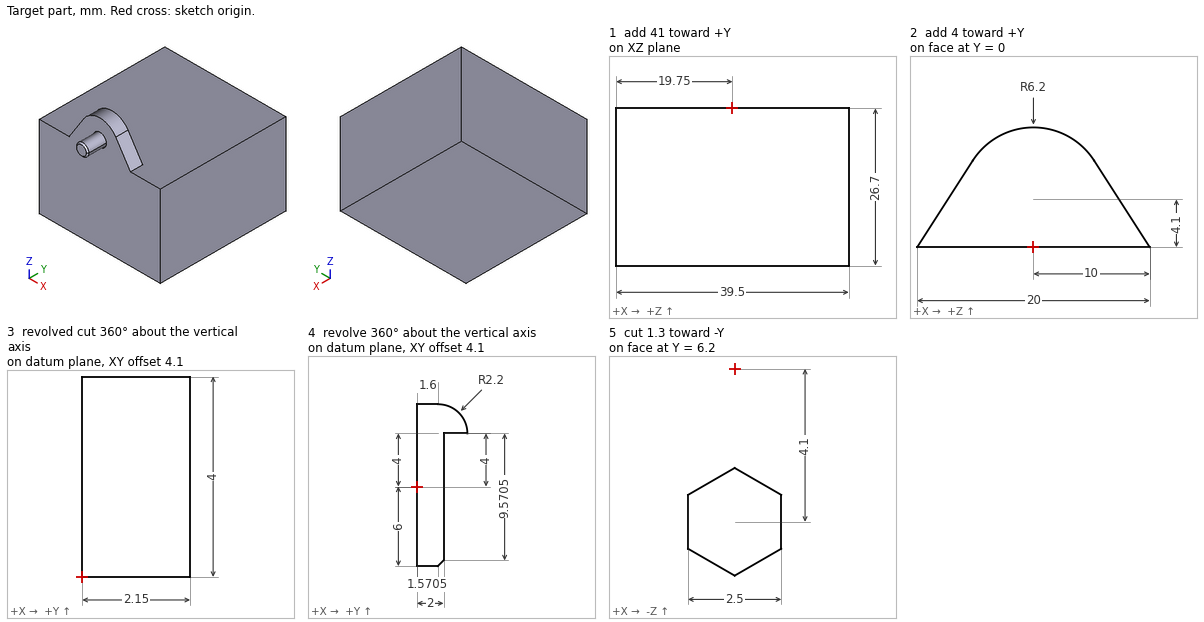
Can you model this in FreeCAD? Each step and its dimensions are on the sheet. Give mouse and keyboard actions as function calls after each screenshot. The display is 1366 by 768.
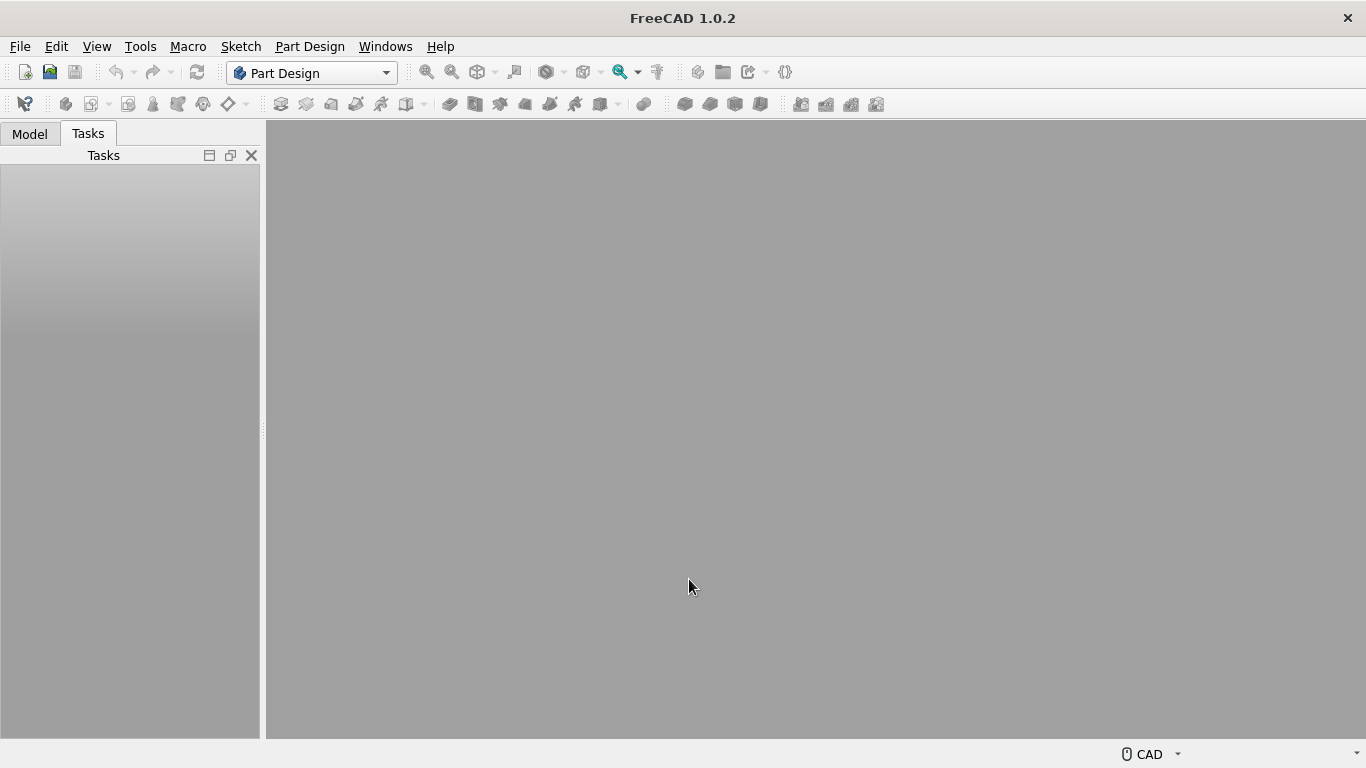
key(ctrl+n)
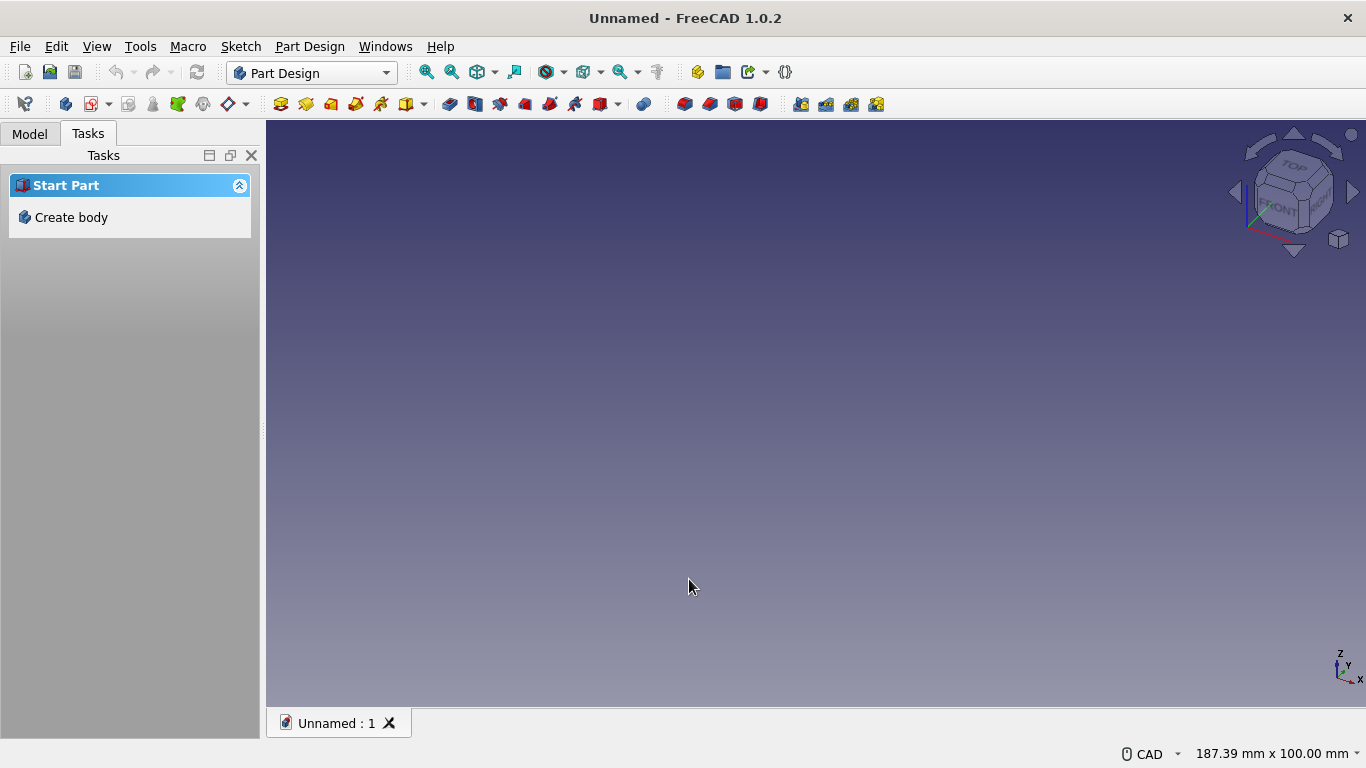
click(90, 104)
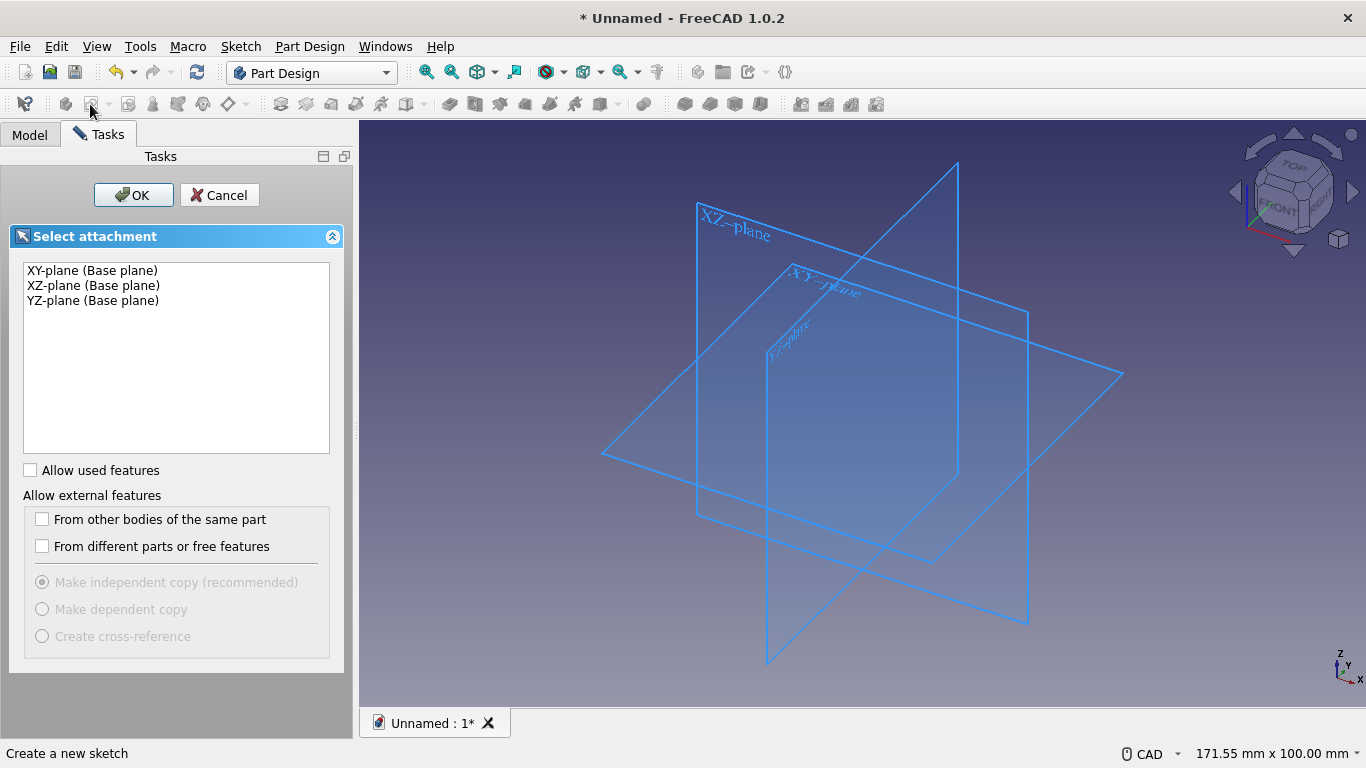
click(84, 286)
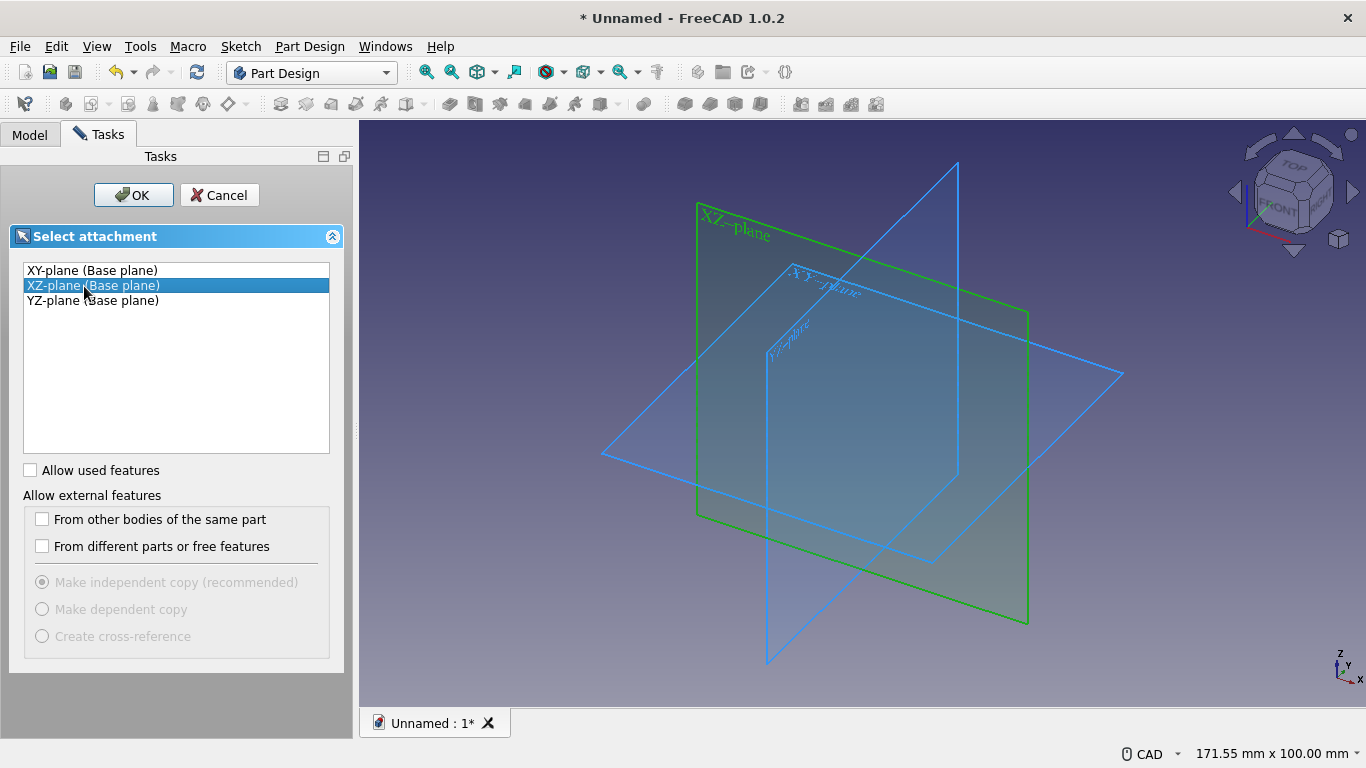
click(134, 195)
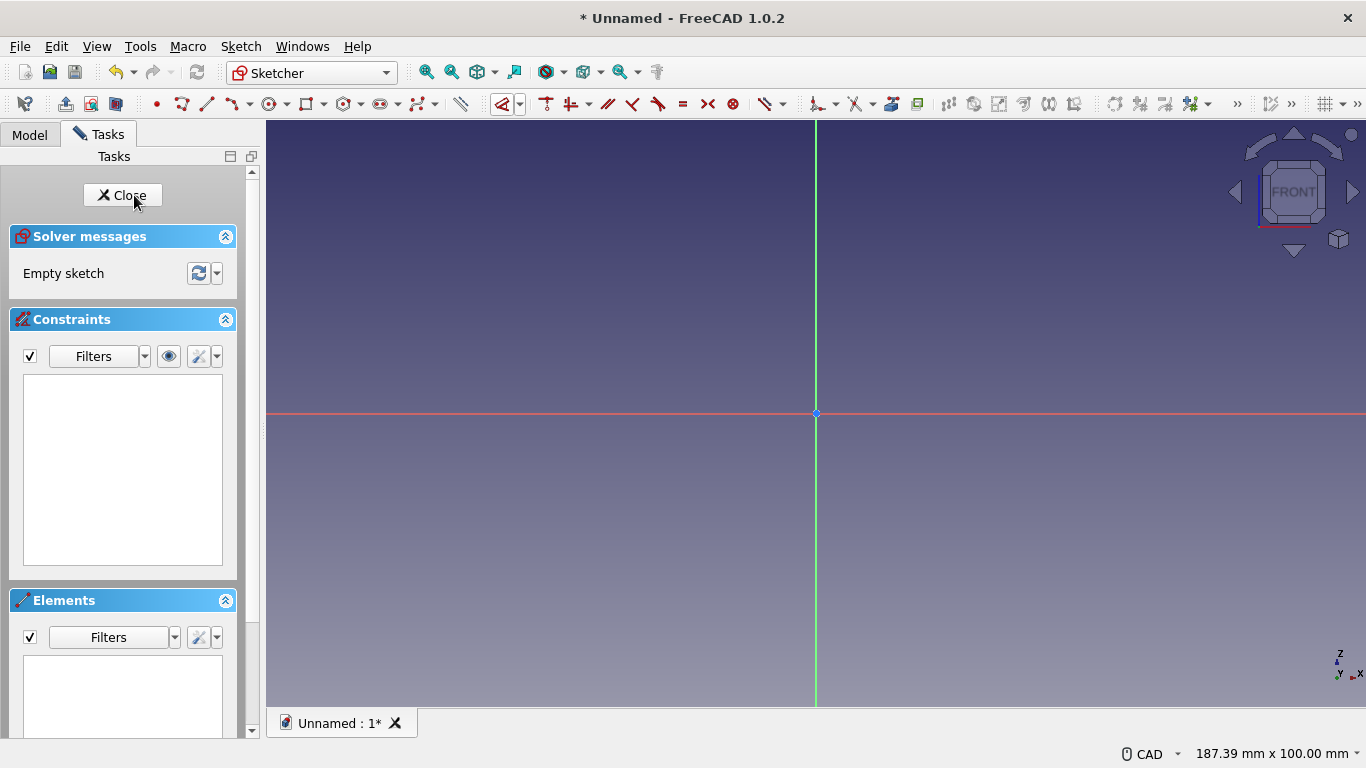
scroll(872, 556, up, 4)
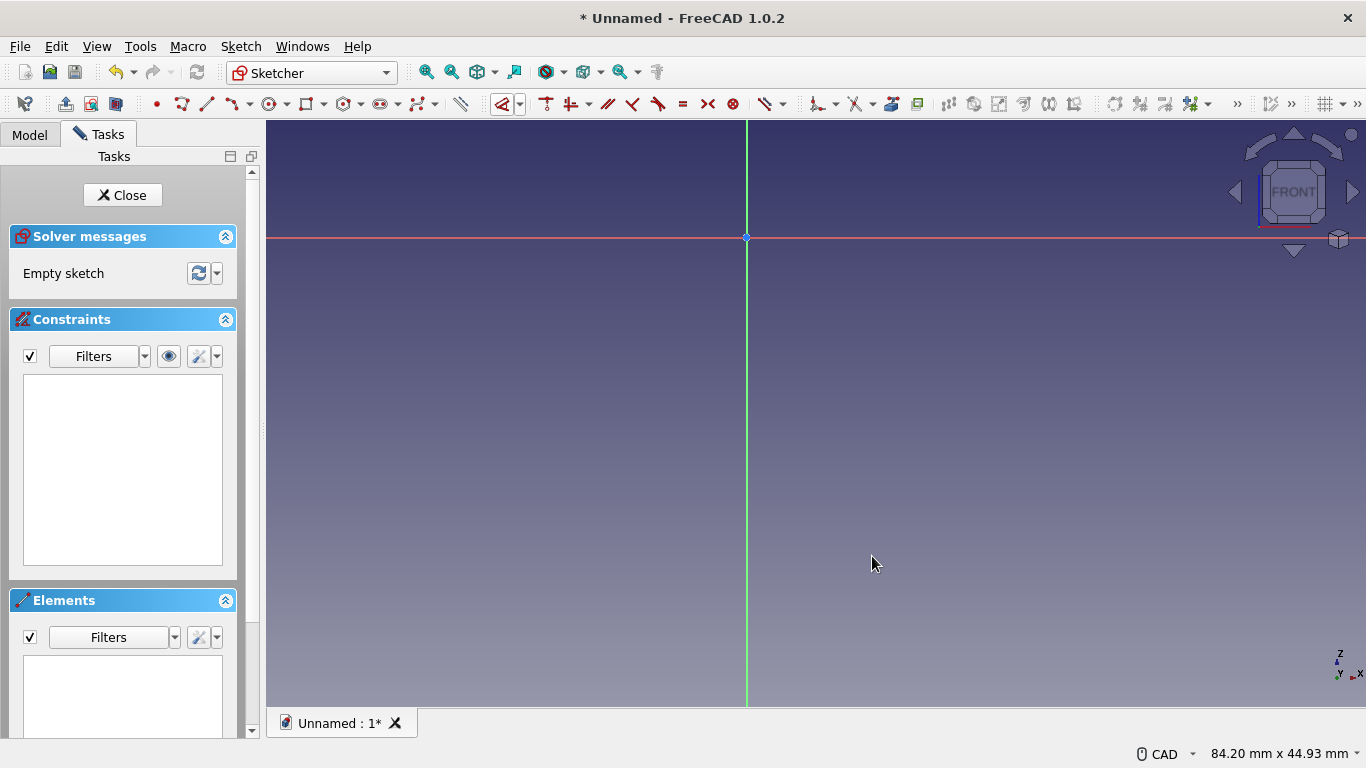
click(306, 104)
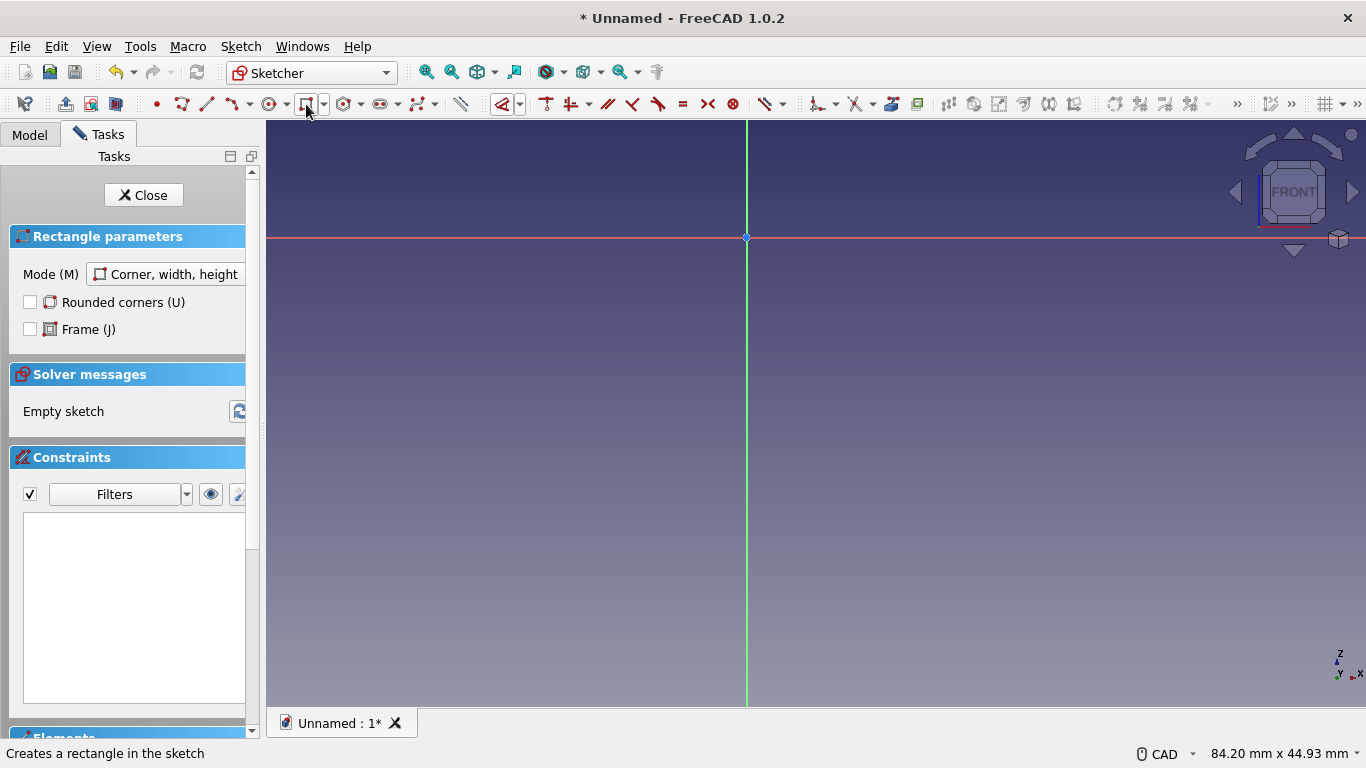
click(489, 238)
move(1005, 587)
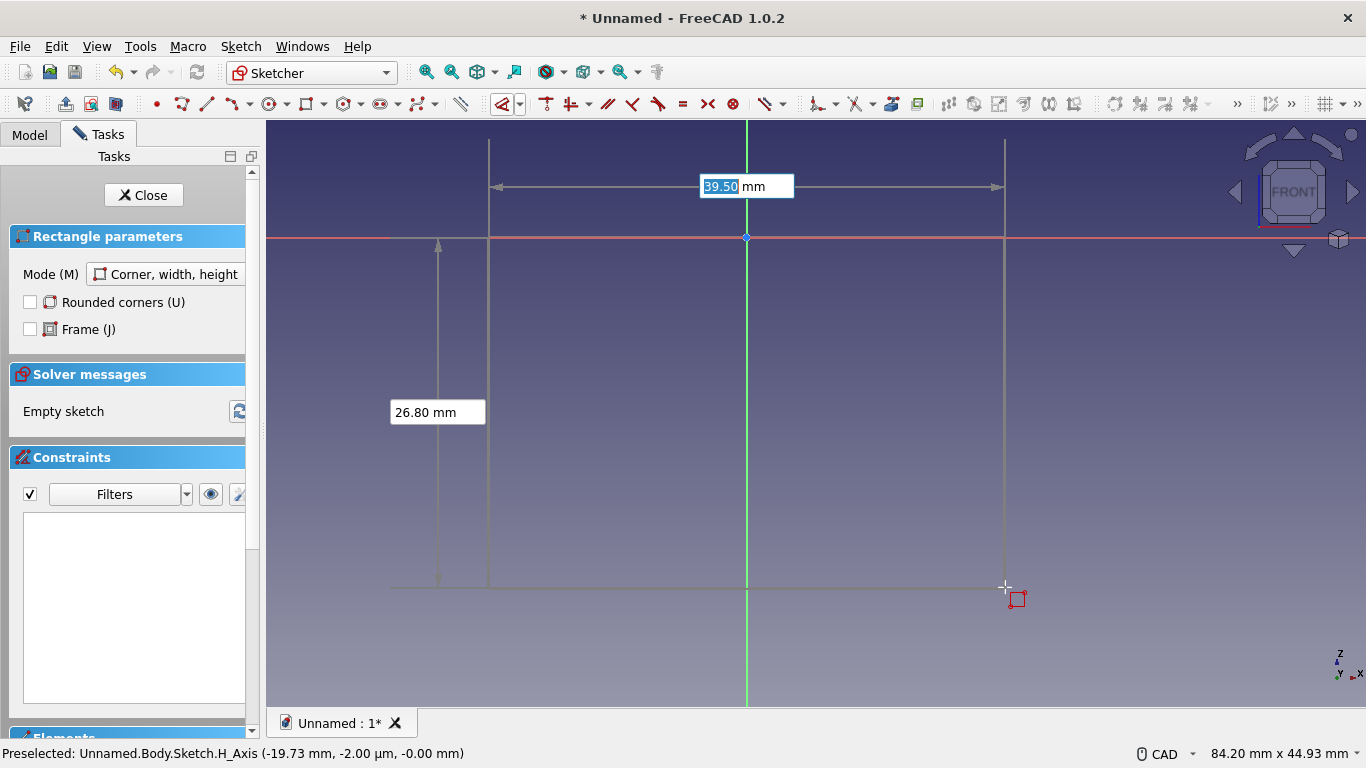
text(39.5)
key(Tab)
text(26.7)
key(Return)
key(Escape)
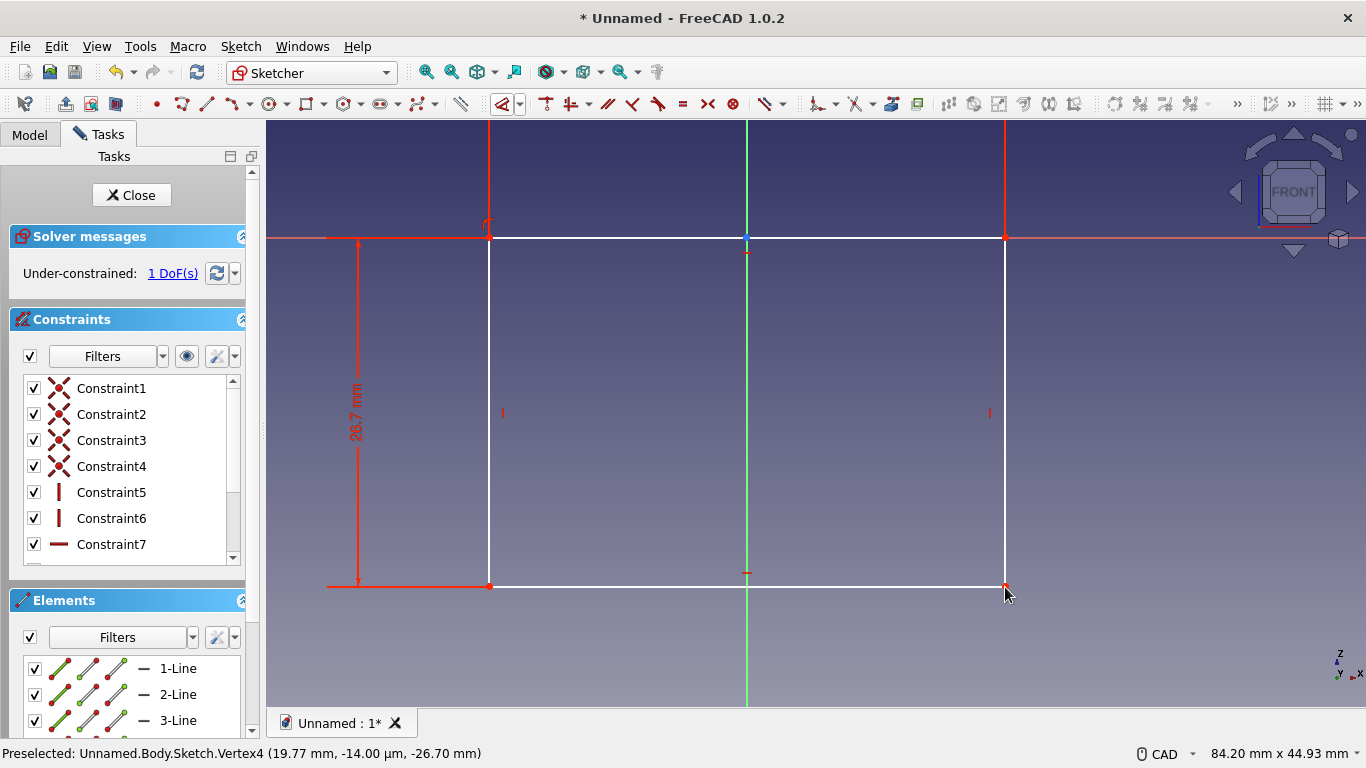
click(489, 238)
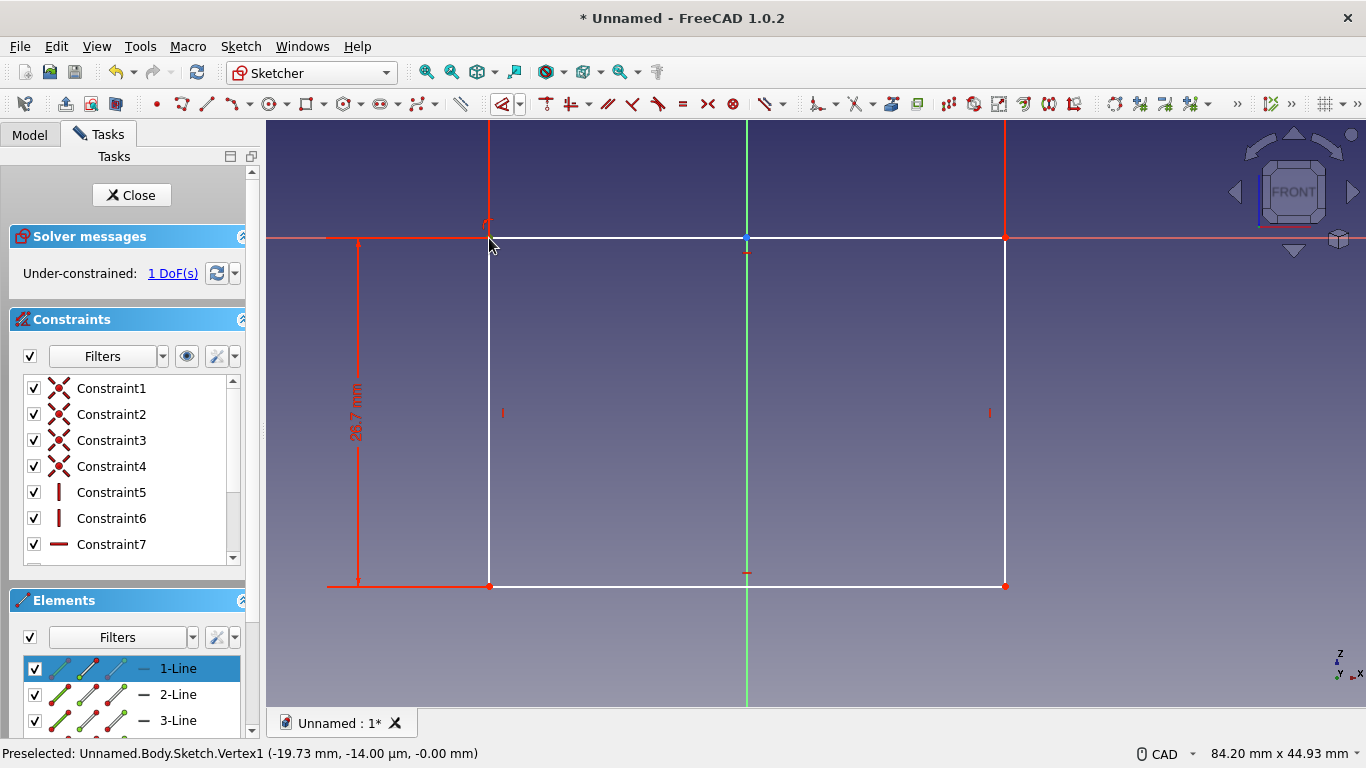
key(l)